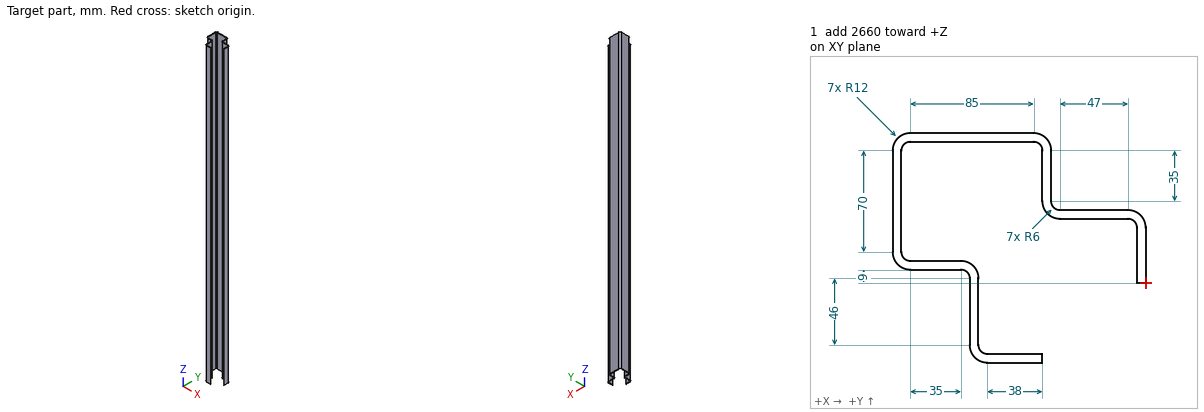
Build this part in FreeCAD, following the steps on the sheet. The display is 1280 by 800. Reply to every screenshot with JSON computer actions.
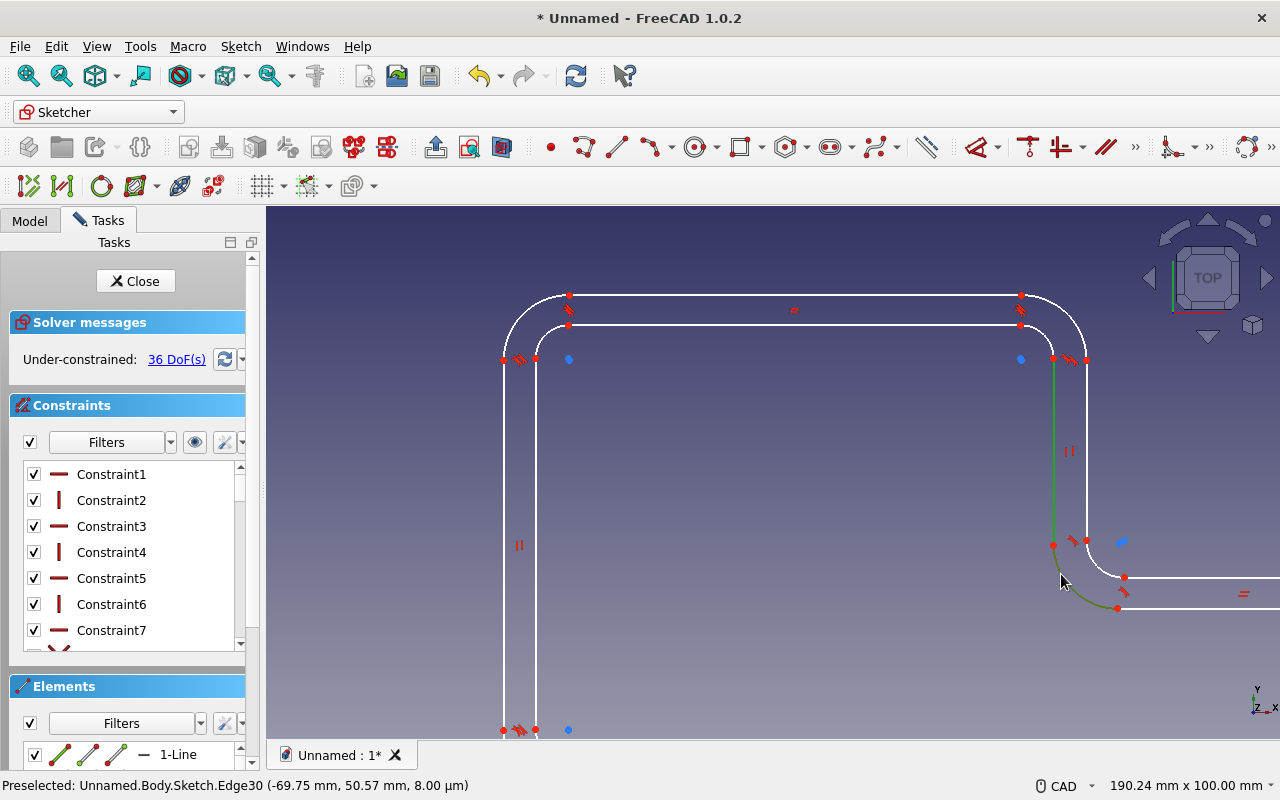
{"action": "key", "text": "t"}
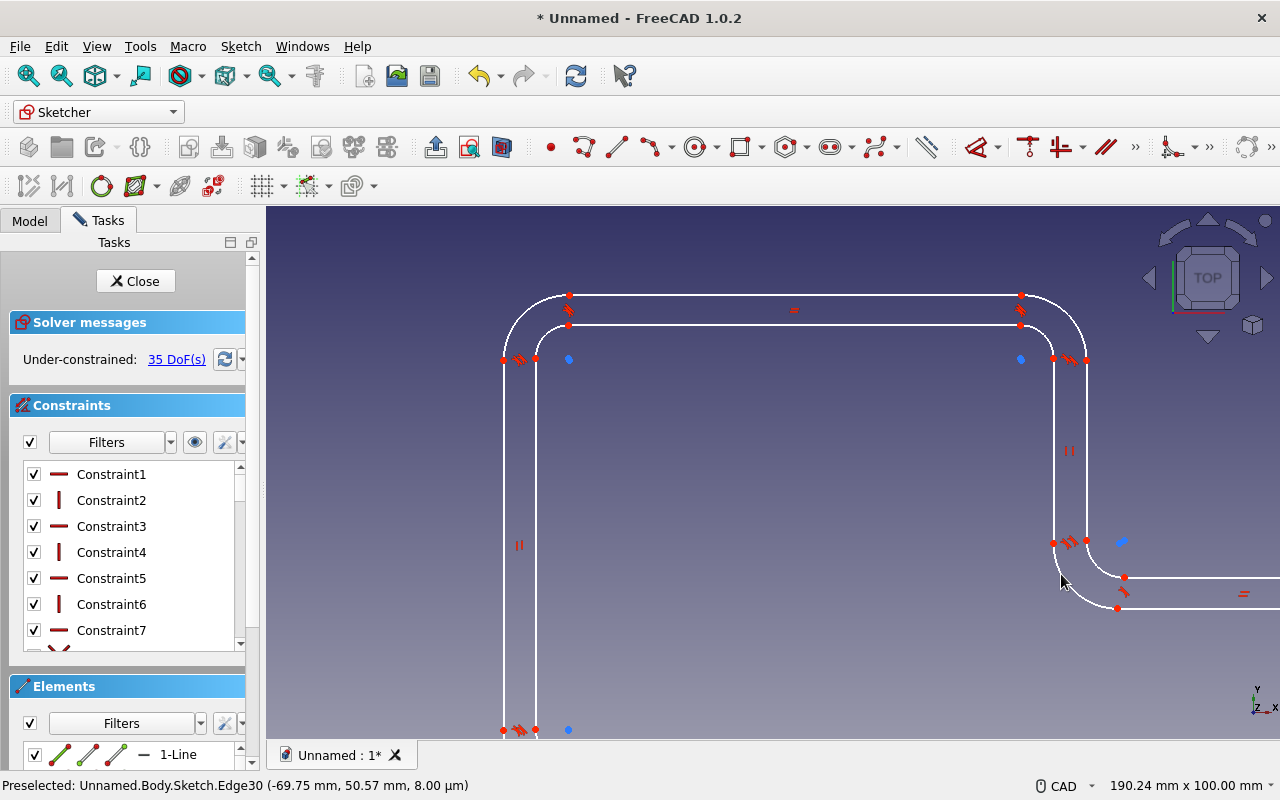
{"action": "scroll", "coordinate": [551, 332], "scroll_direction": "down", "scroll_amount": 5}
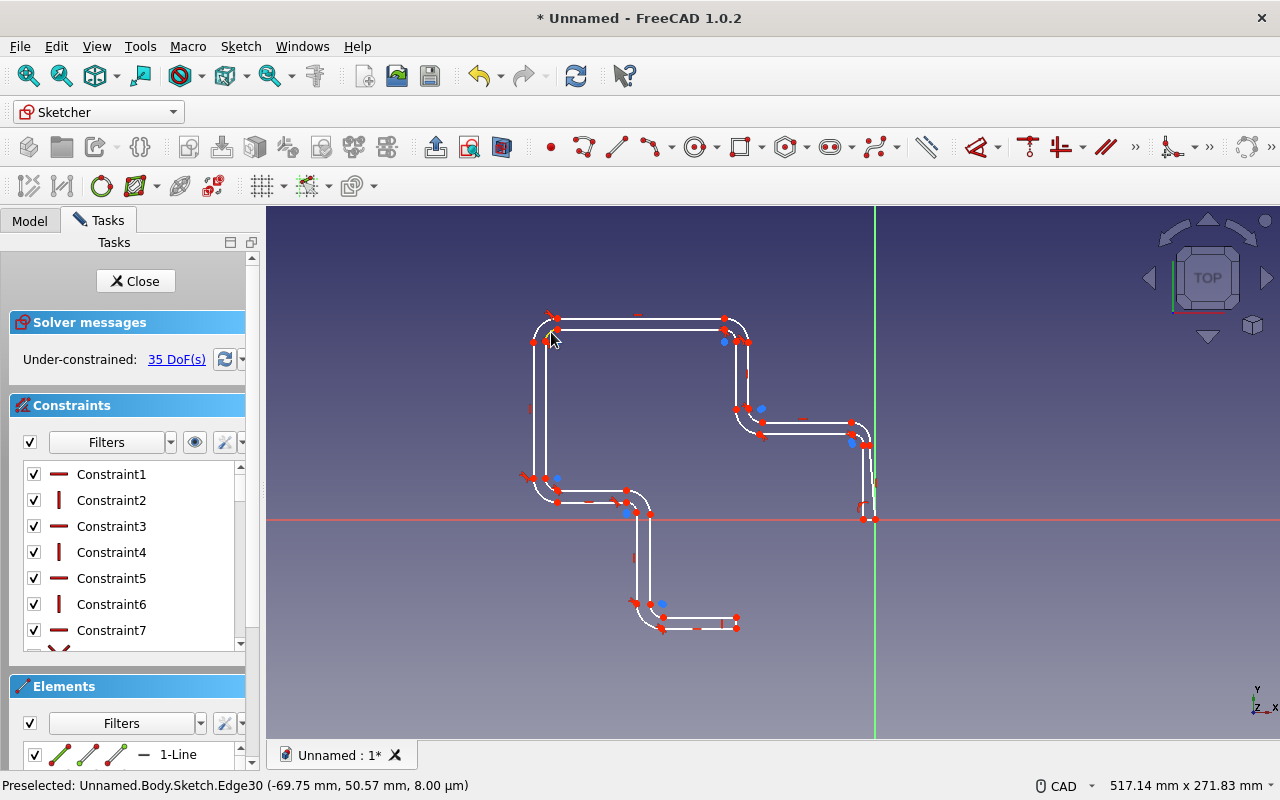
{"action": "left_click", "coordinate": [787, 434]}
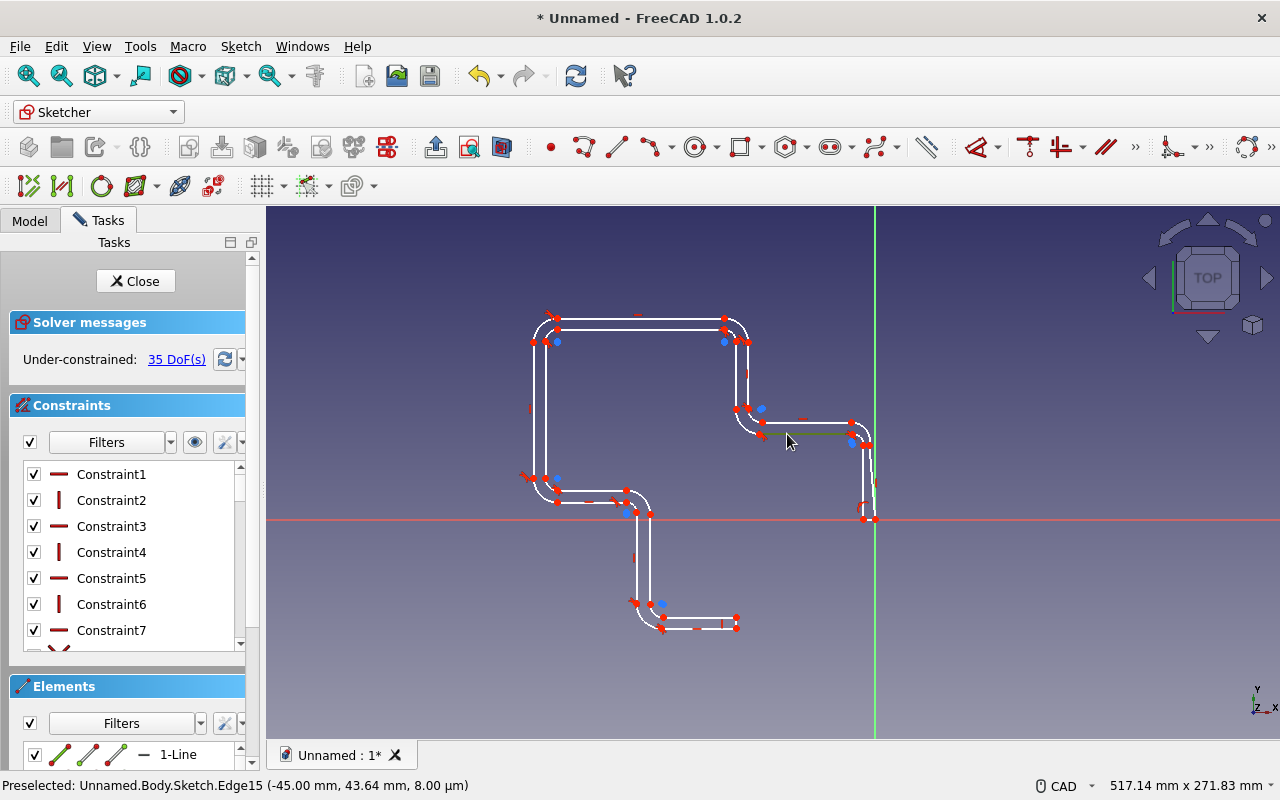
{"action": "scroll", "coordinate": [739, 421], "scroll_direction": "up", "scroll_amount": 2}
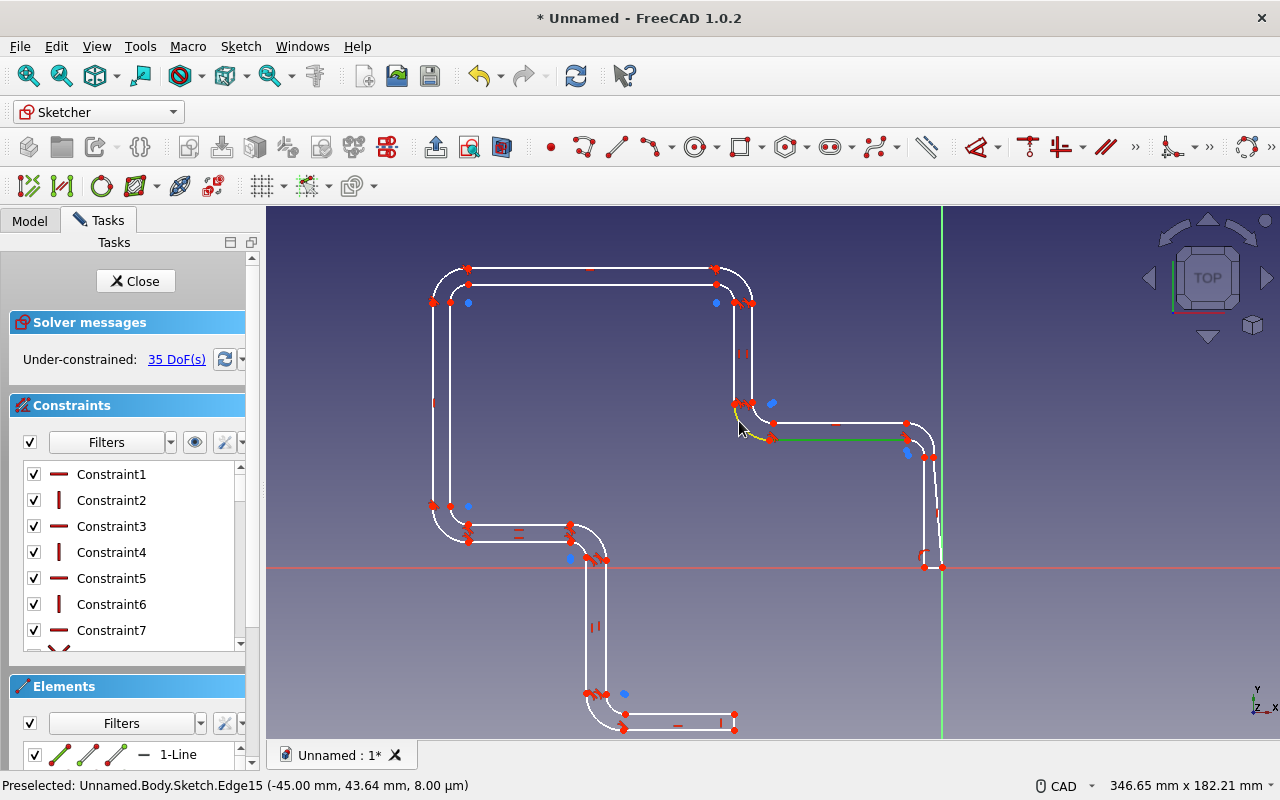
{"action": "left_click", "coordinate": [738, 420]}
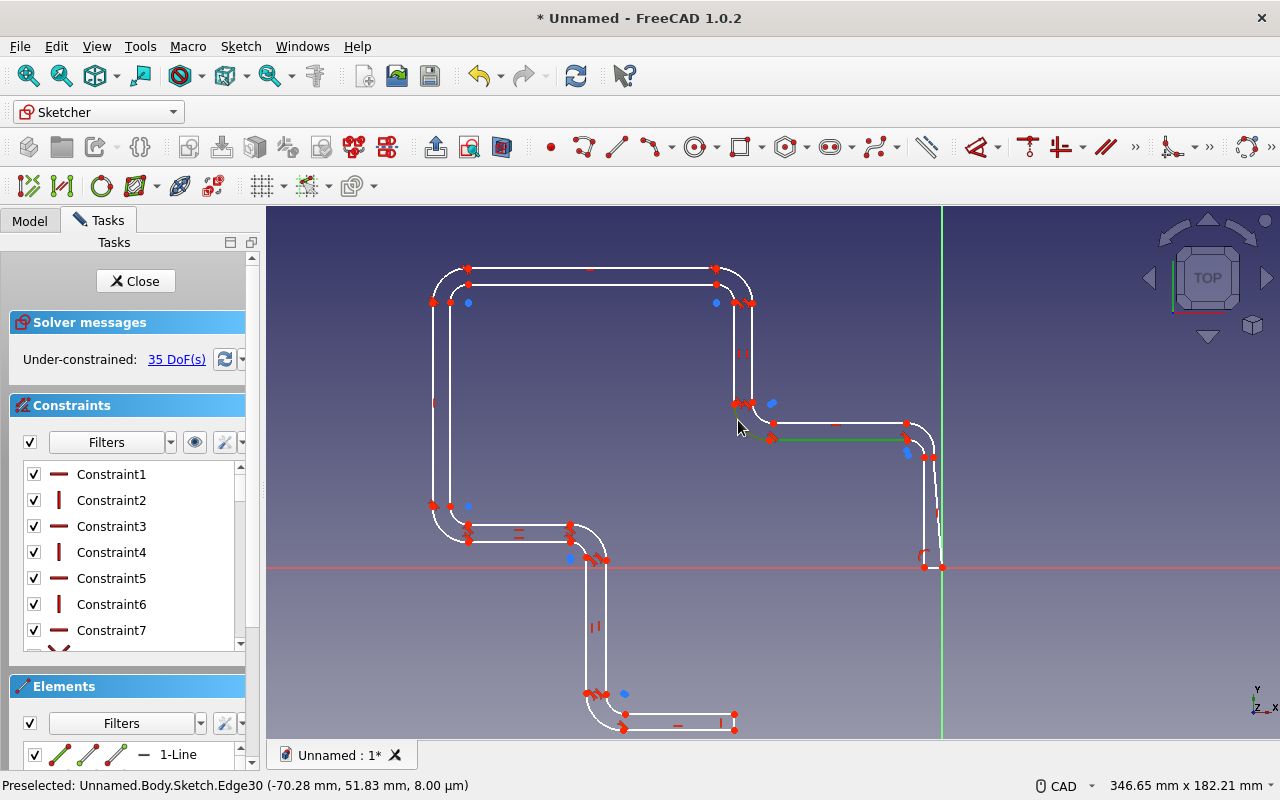
{"action": "key", "text": "t"}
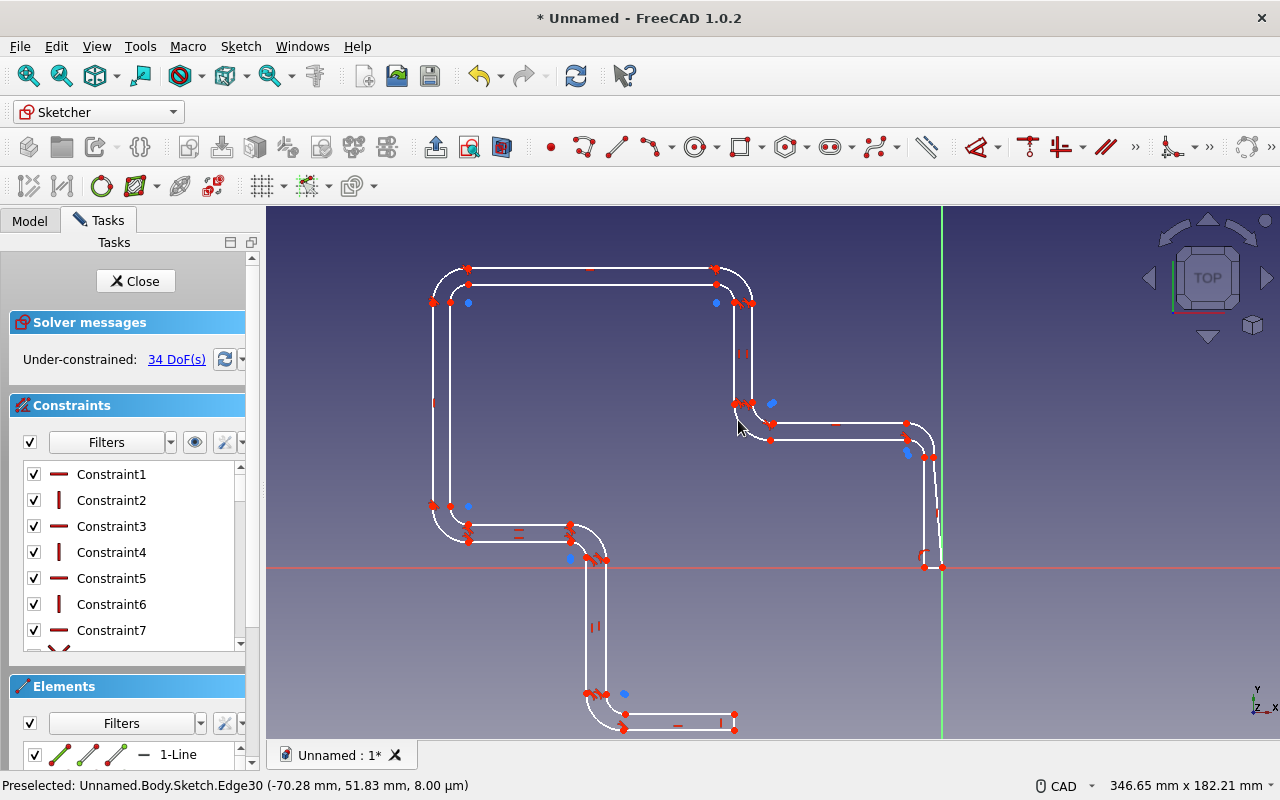
{"action": "left_click", "coordinate": [811, 440]}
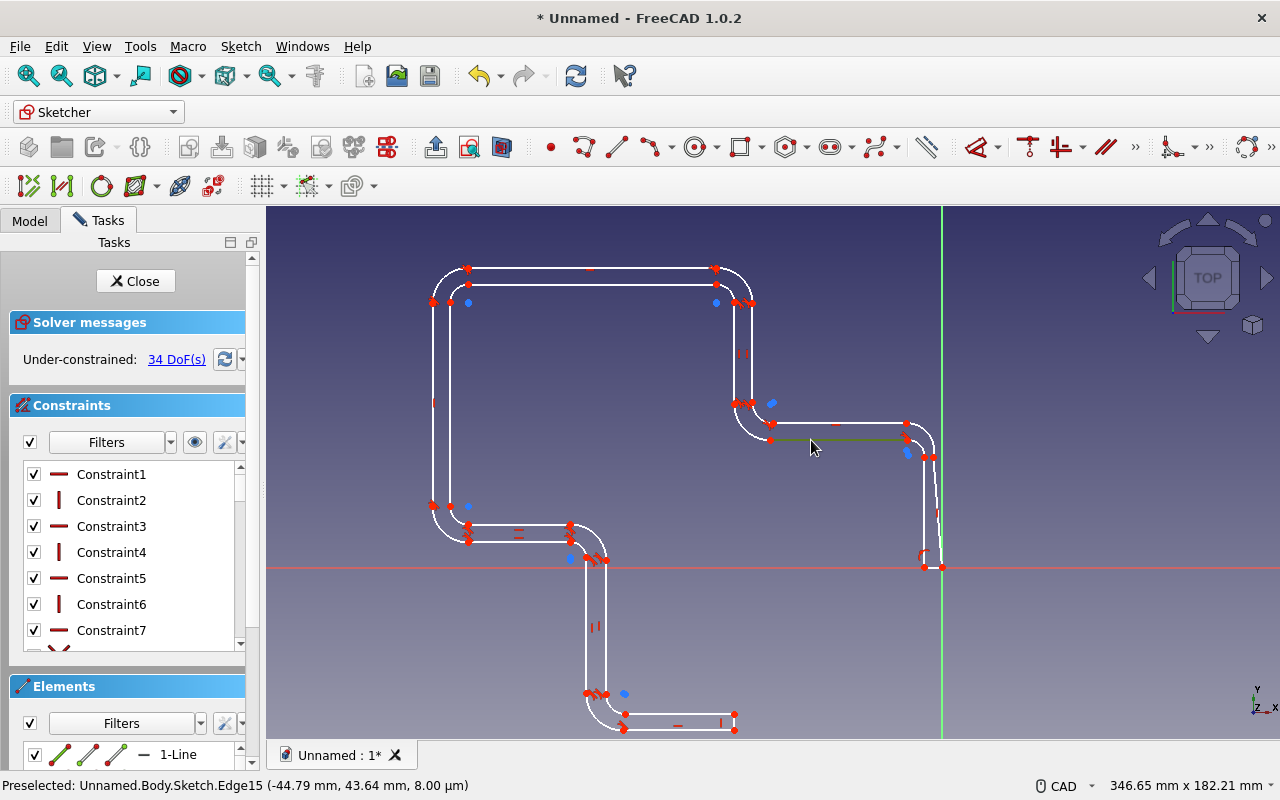
{"action": "left_click", "coordinate": [920, 445]}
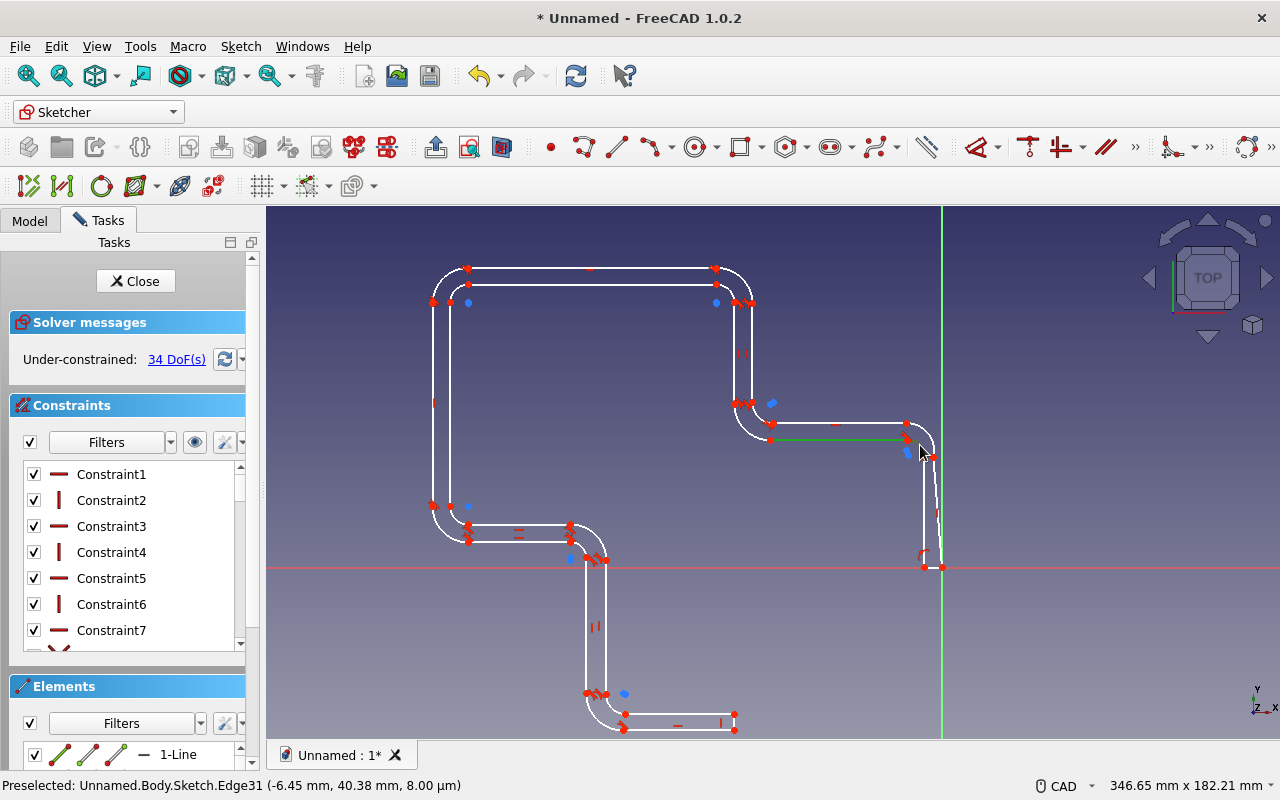
{"action": "key", "text": "t"}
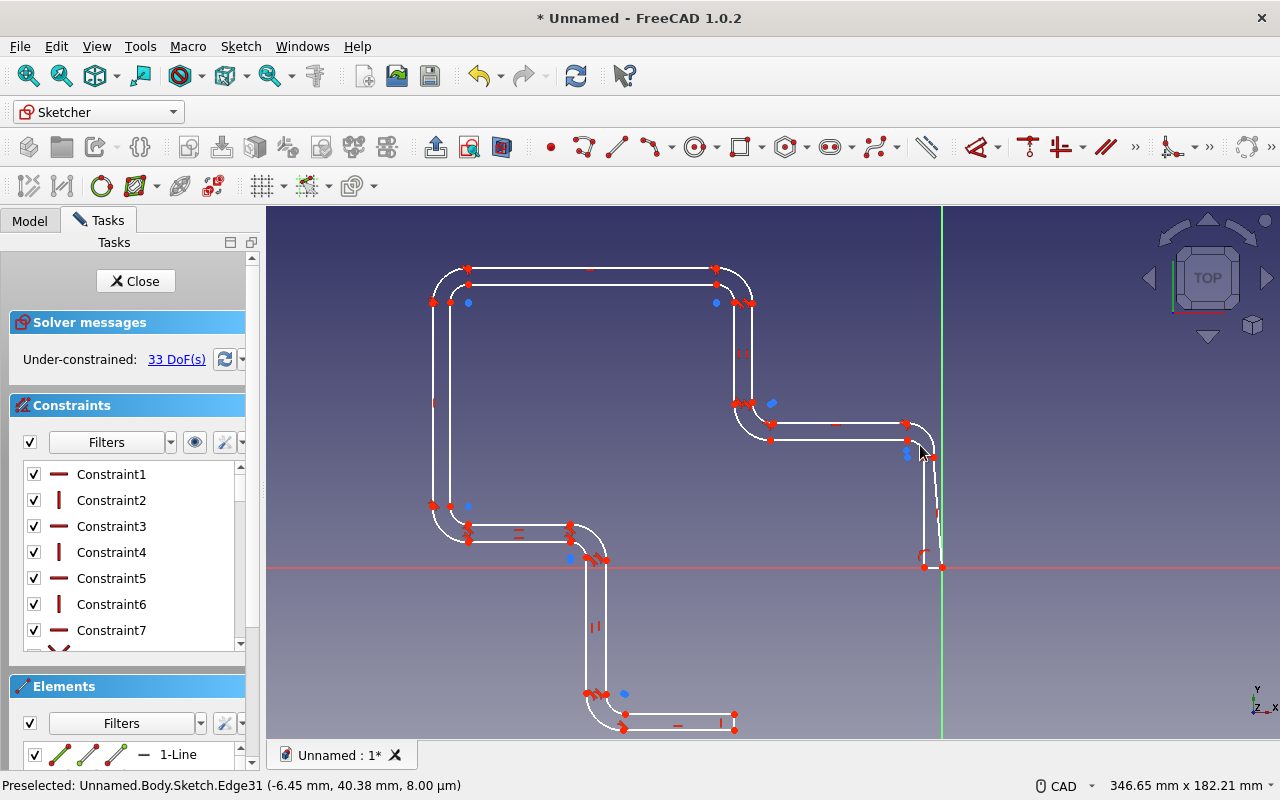
{"action": "left_click", "coordinate": [924, 490]}